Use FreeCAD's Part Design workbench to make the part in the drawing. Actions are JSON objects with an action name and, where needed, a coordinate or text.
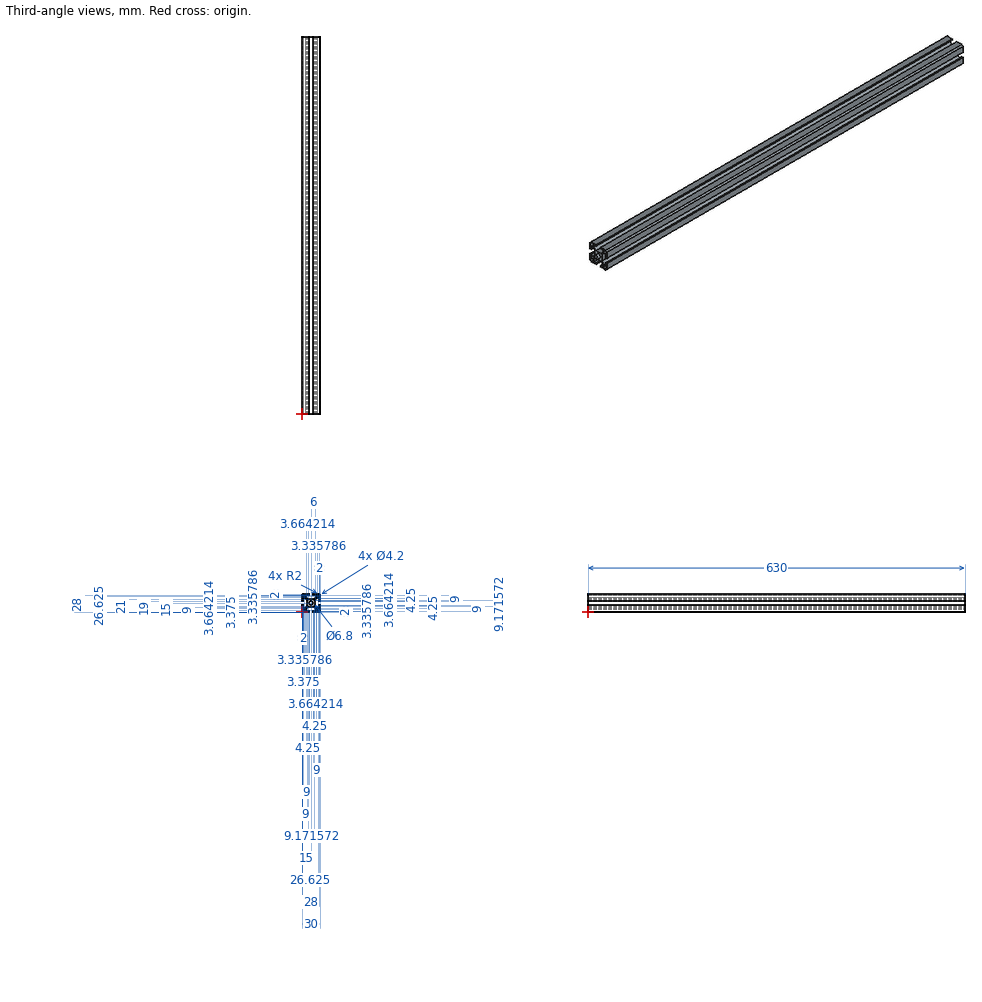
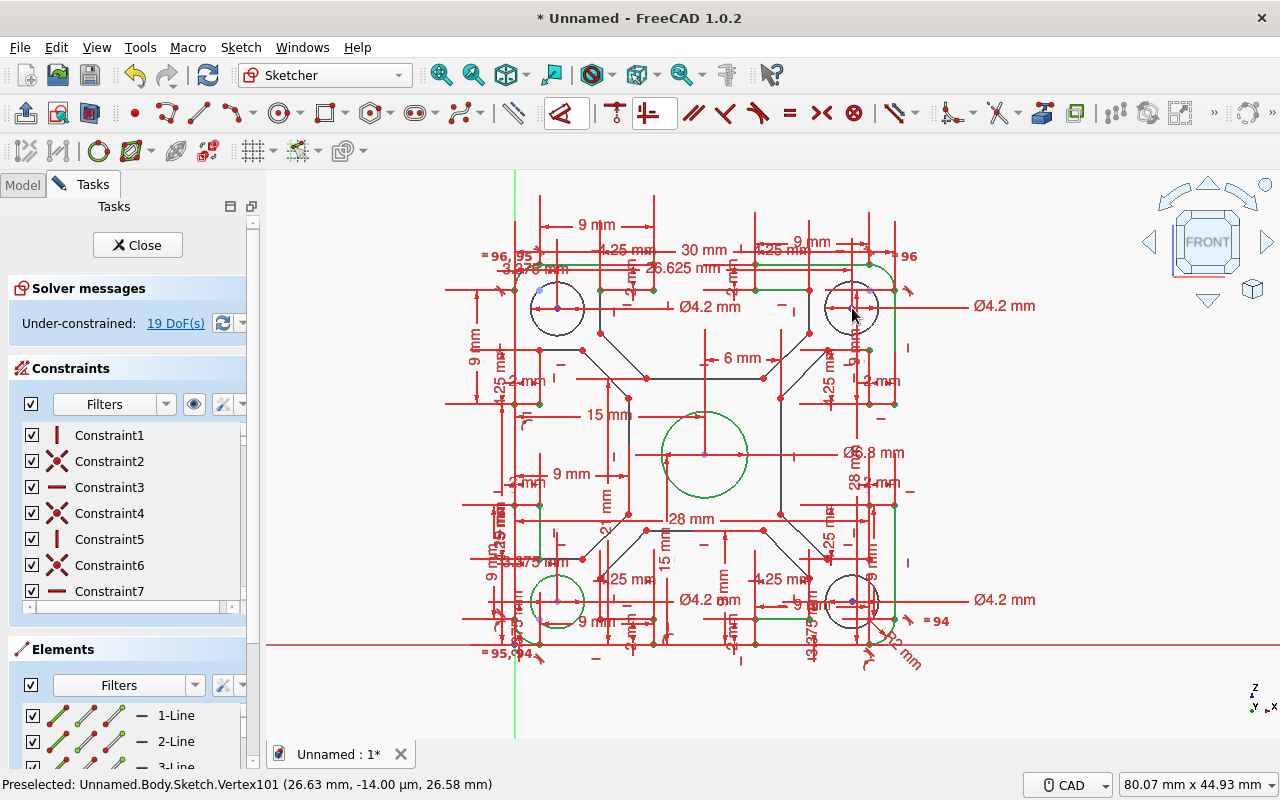
{"action": "left_click", "coordinate": [852, 308]}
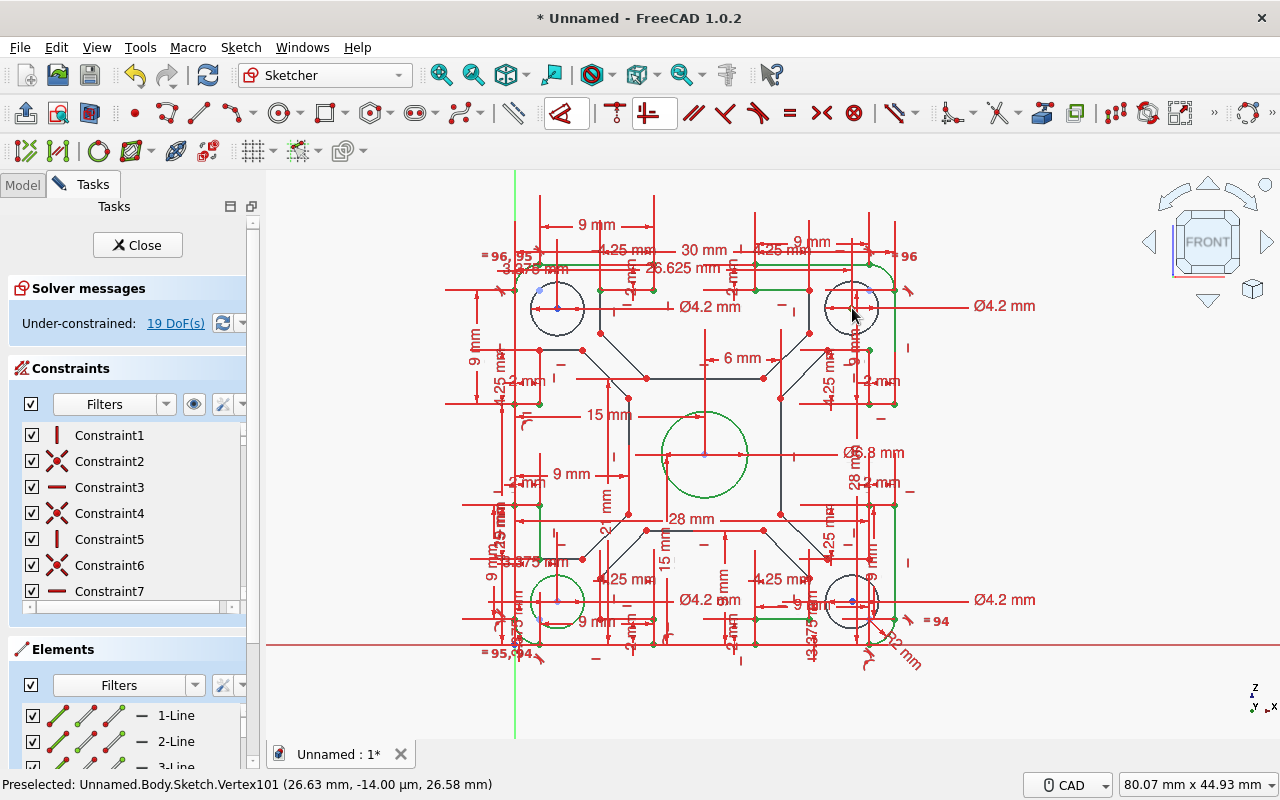
{"action": "key", "text": "i"}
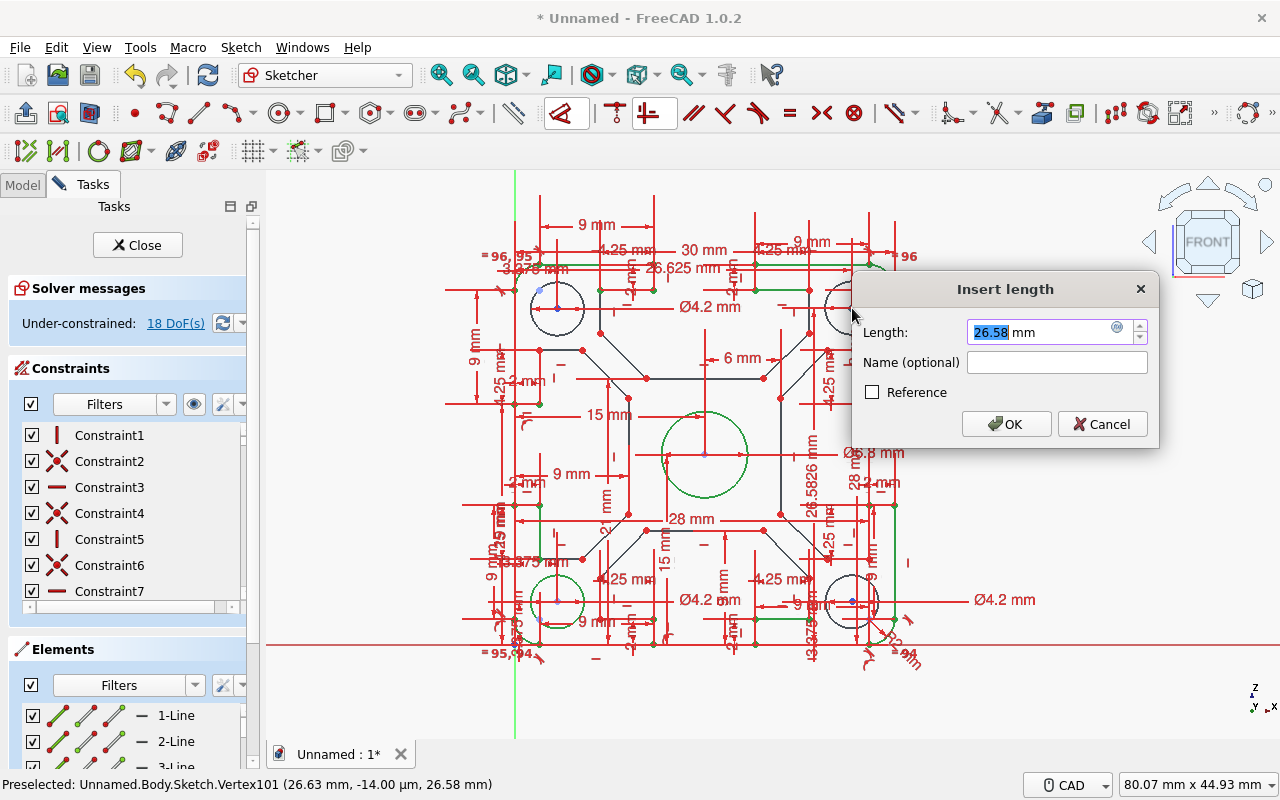
{"action": "type", "text": "26.625"}
{"action": "key", "text": "Return"}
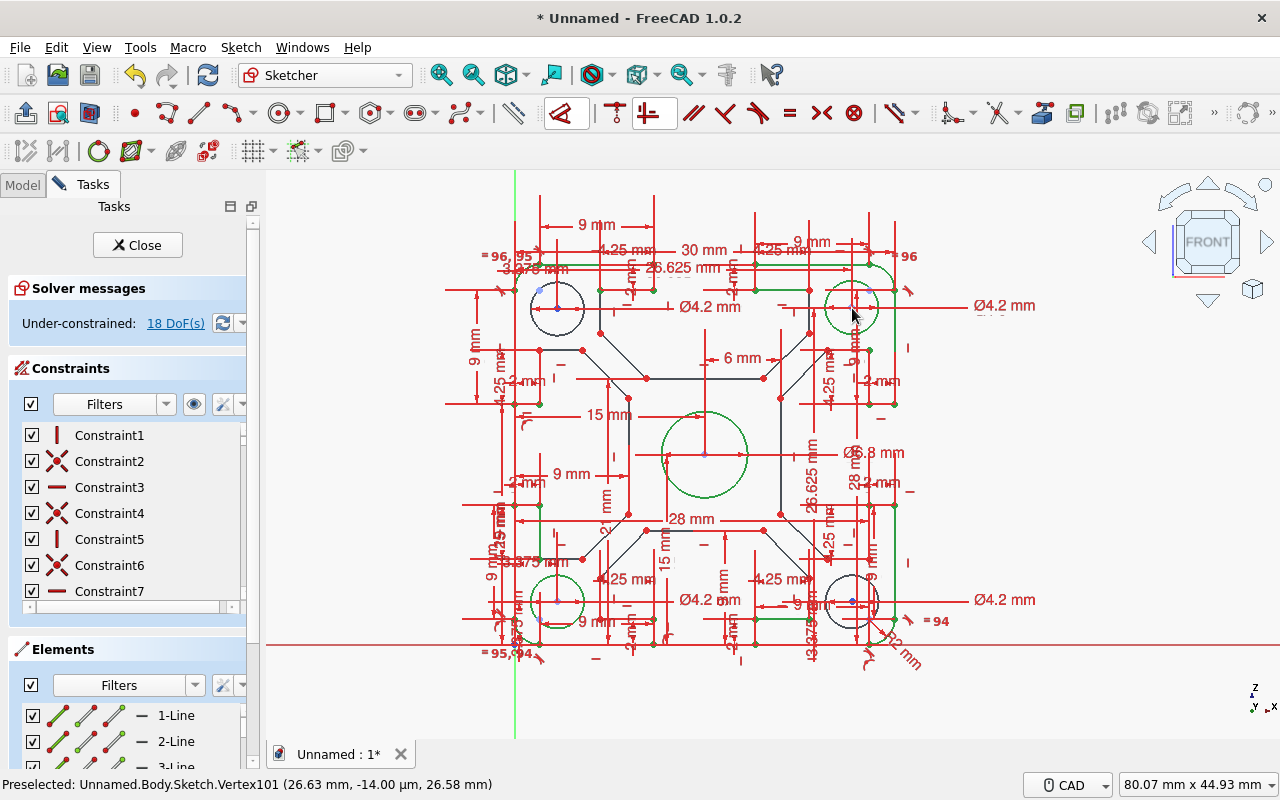
{"action": "left_click", "coordinate": [557, 309]}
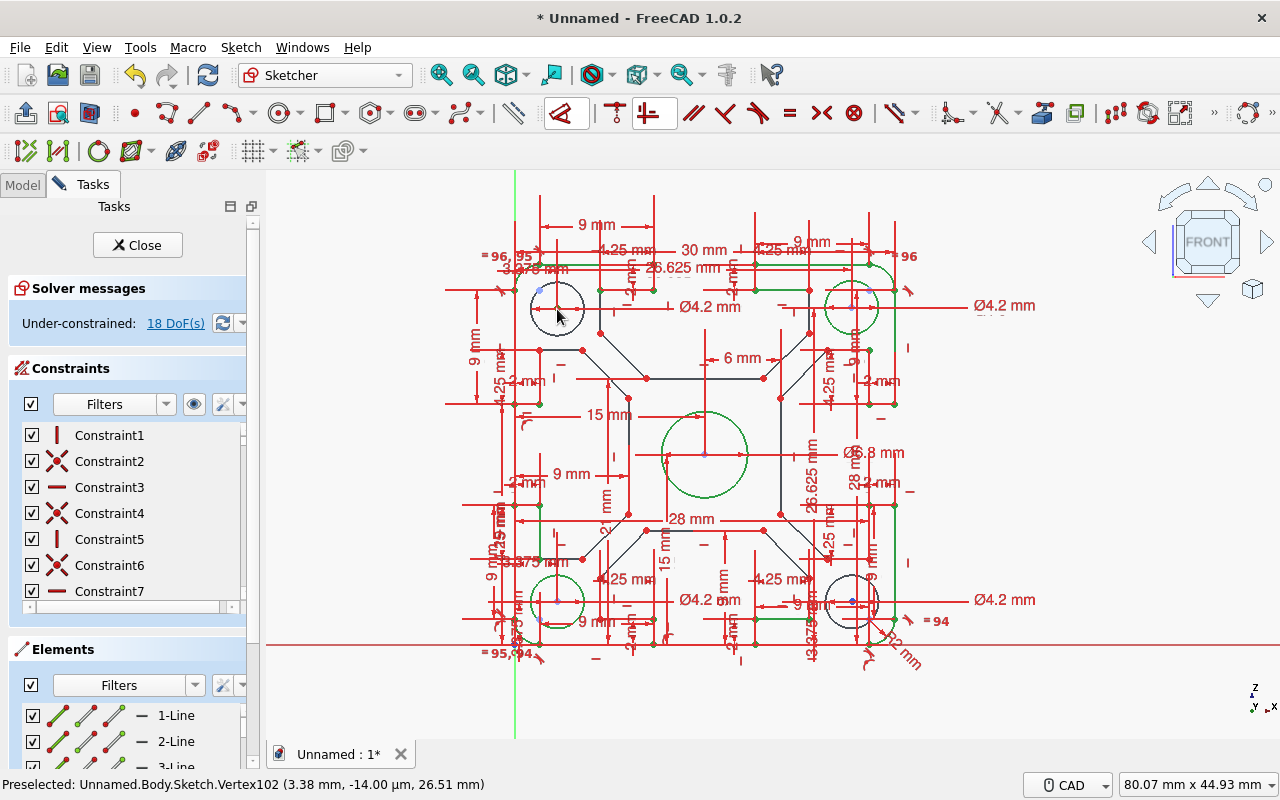
{"action": "key", "text": "i"}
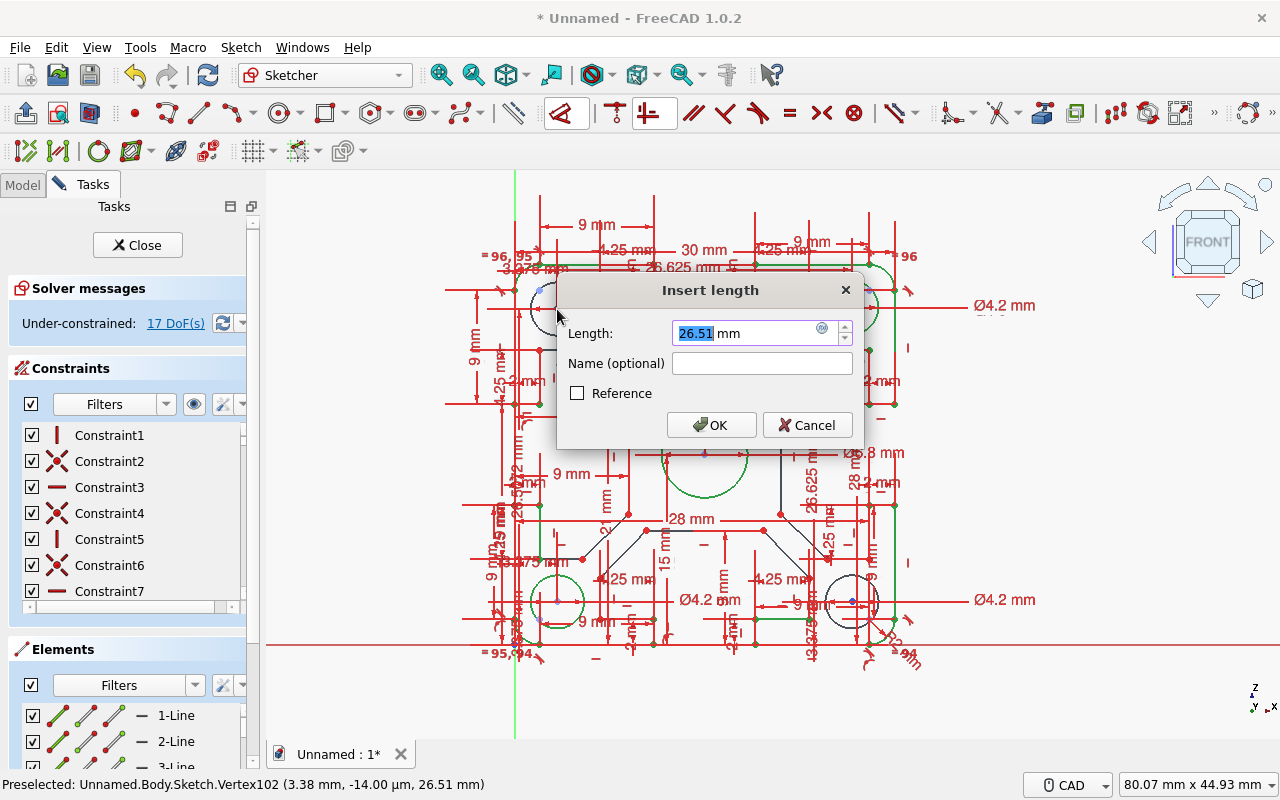
{"action": "type", "text": "26.625"}
{"action": "key", "text": "Return"}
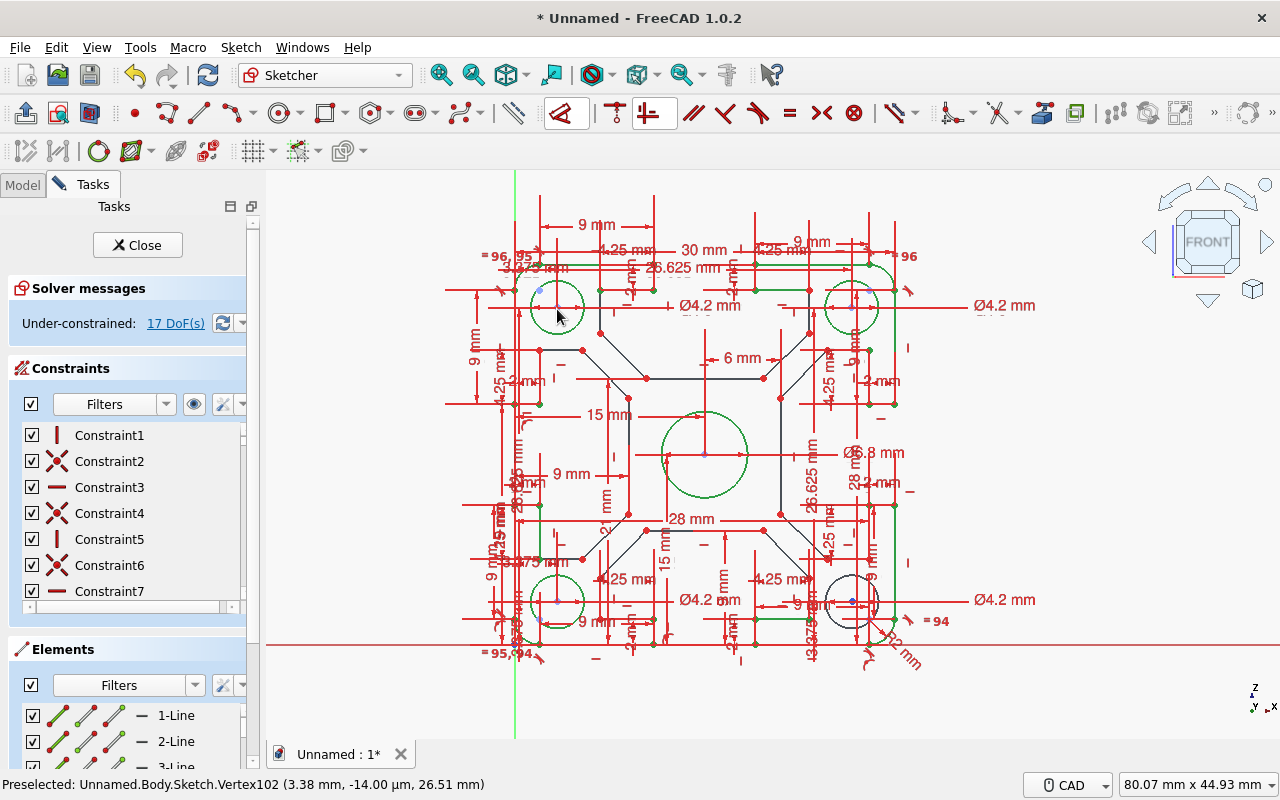
{"action": "left_click", "coordinate": [852, 602]}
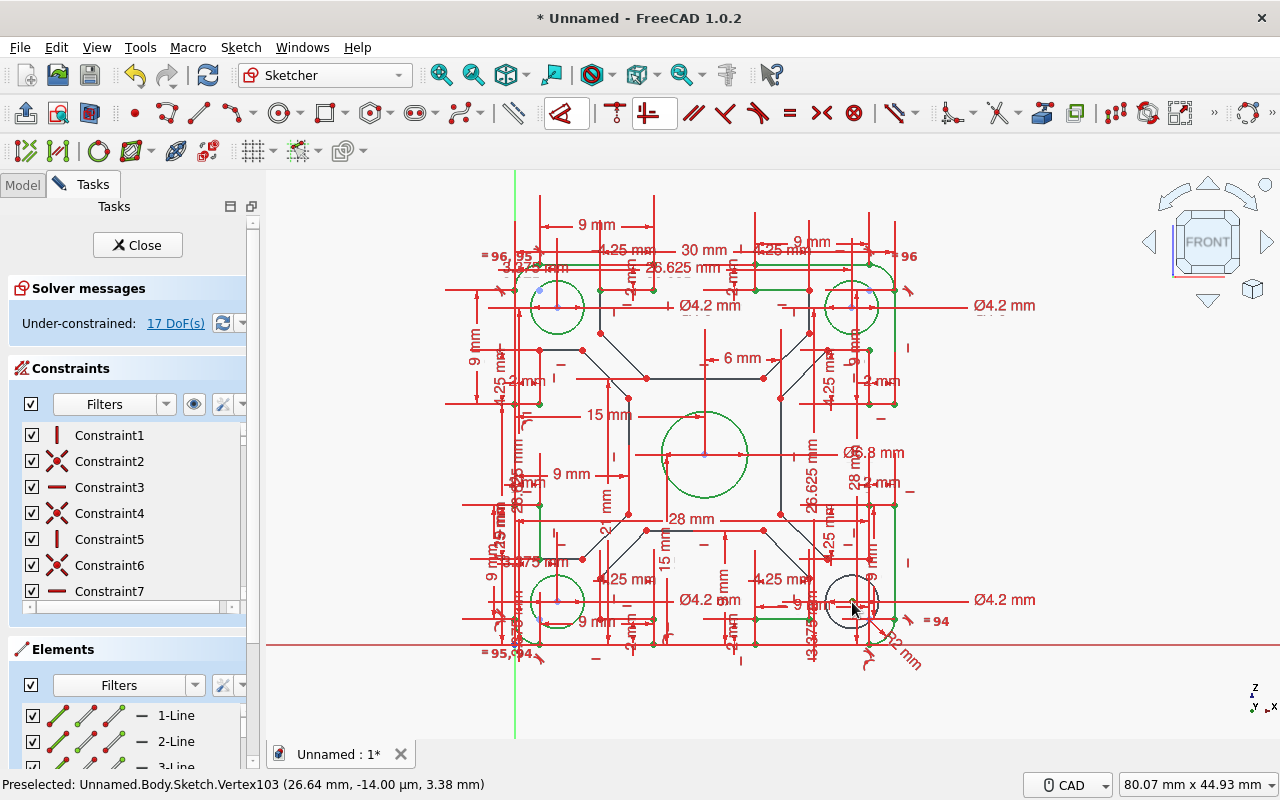
{"action": "key", "text": "l"}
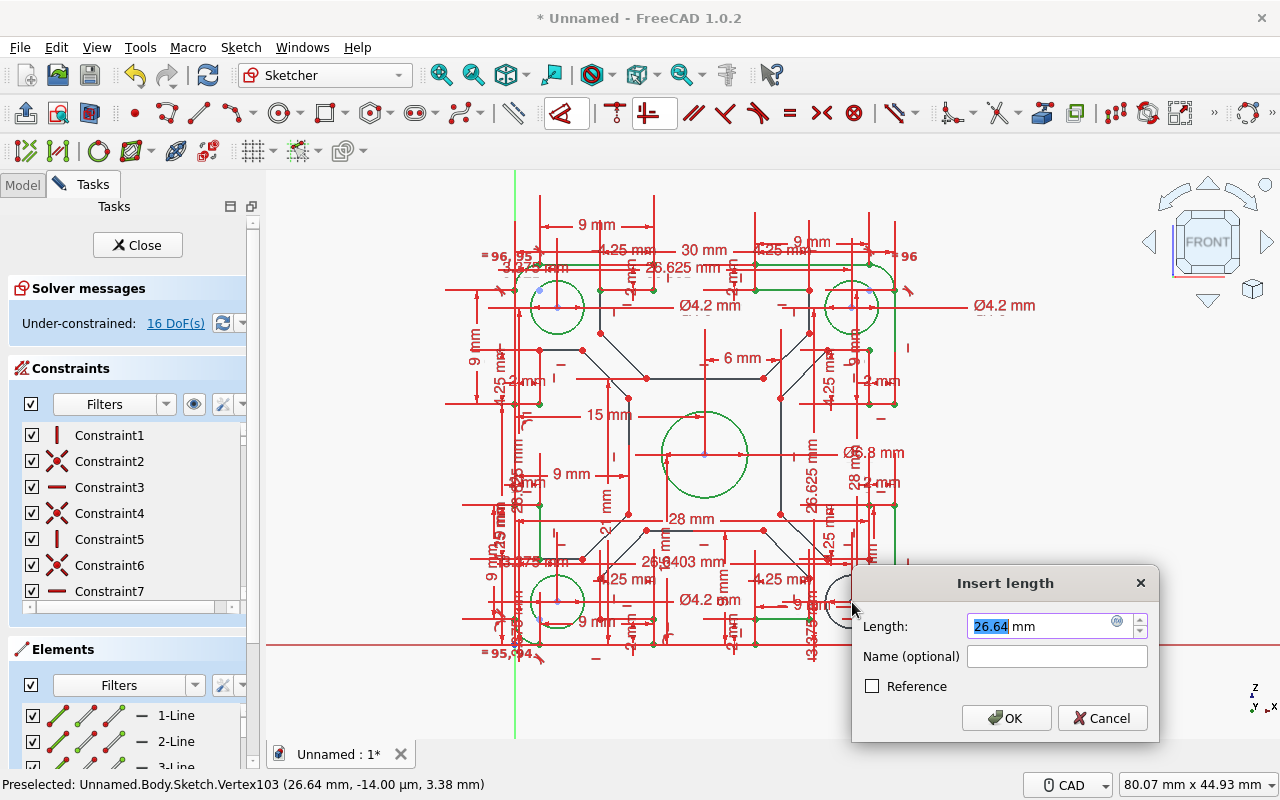
{"action": "type", "text": "26.625"}
{"action": "key", "text": "Return"}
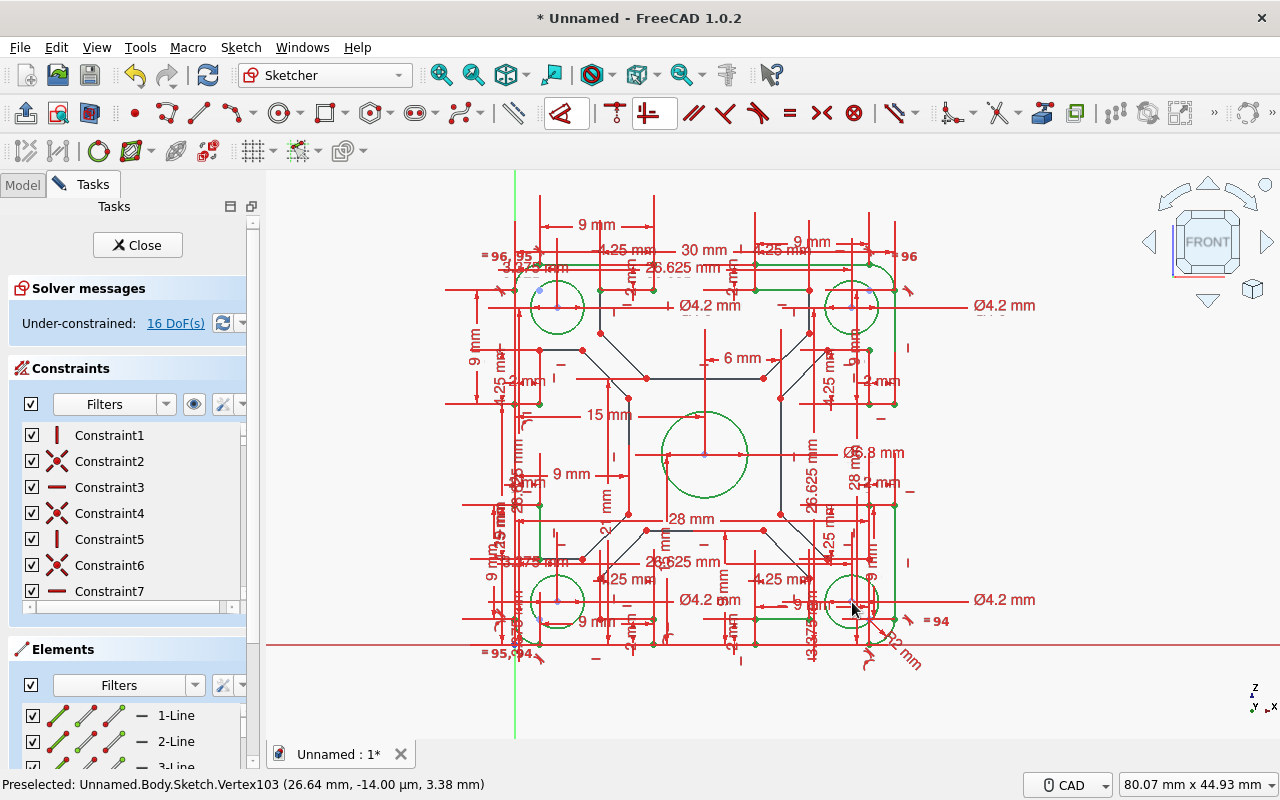
{"action": "left_click", "coordinate": [840, 350]}